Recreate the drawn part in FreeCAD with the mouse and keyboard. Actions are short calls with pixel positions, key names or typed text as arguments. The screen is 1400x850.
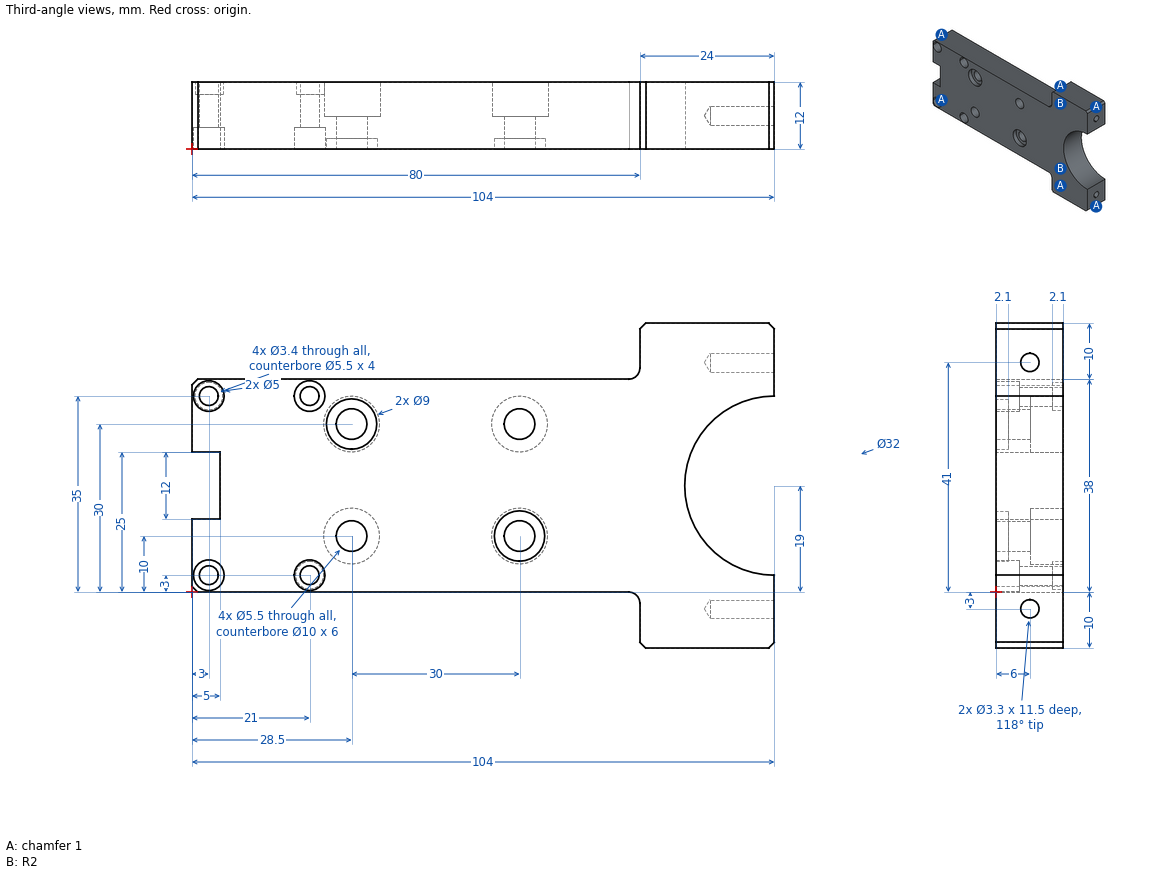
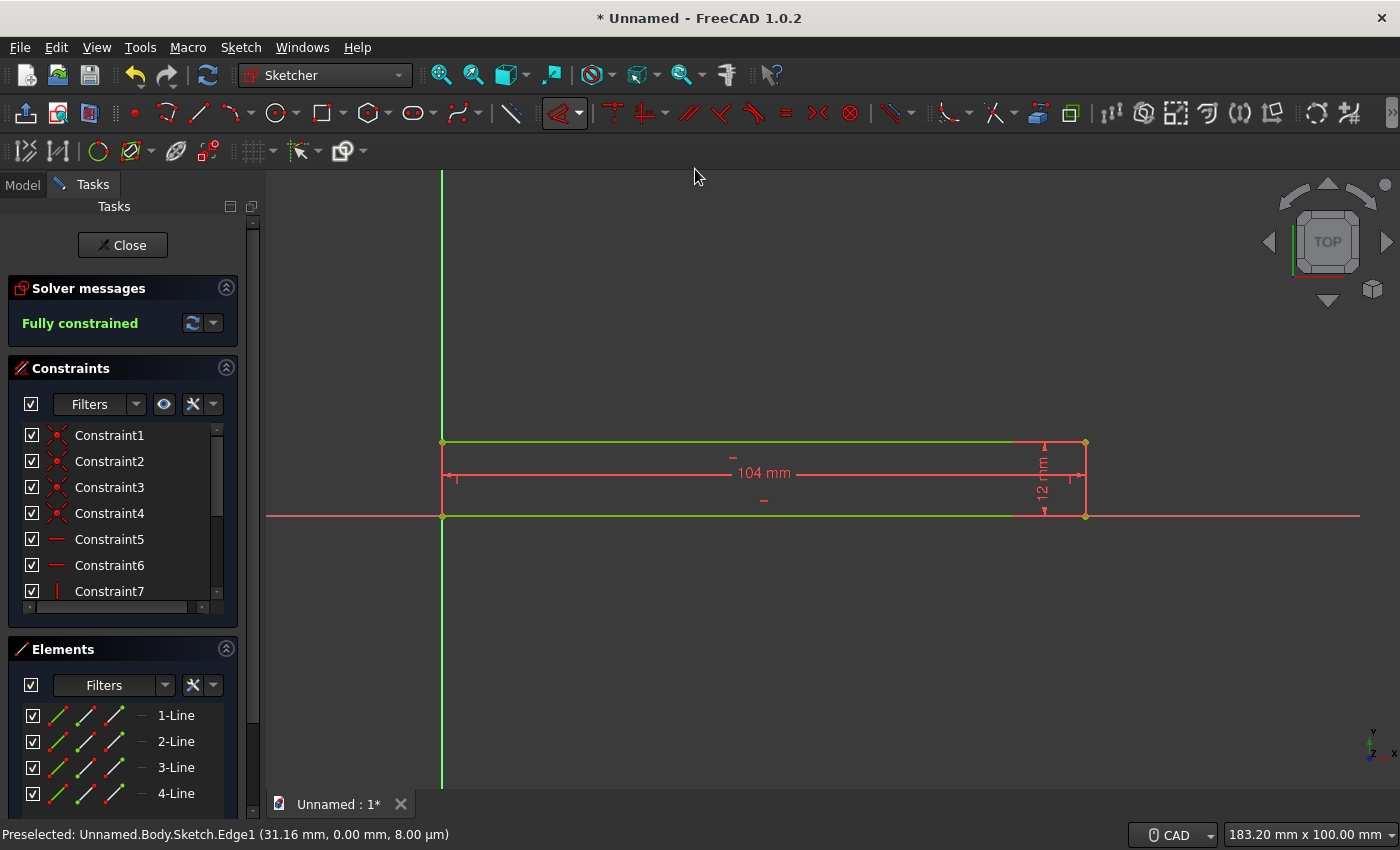
click(123, 245)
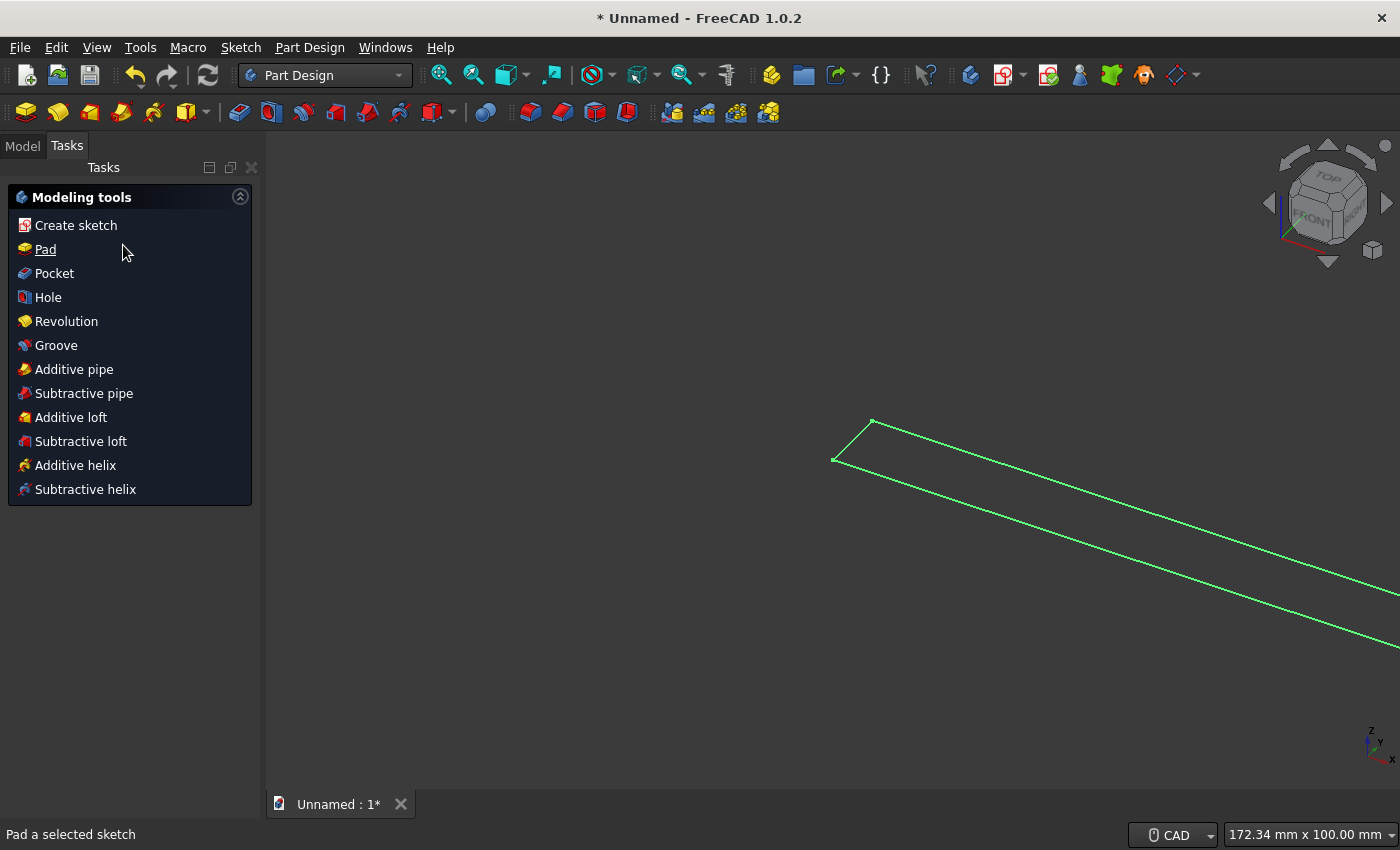
click(26, 112)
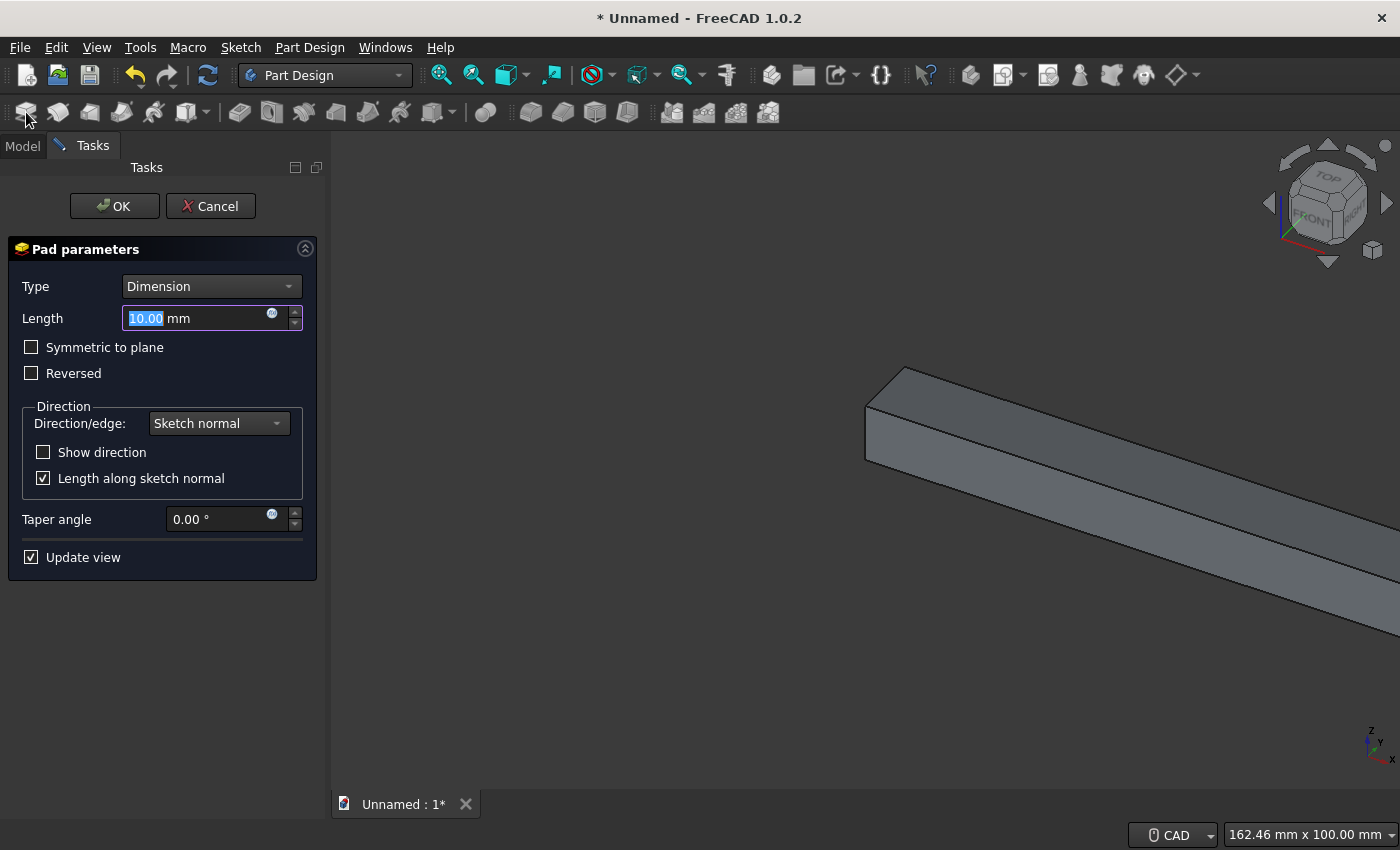
text(38)
key(Tab)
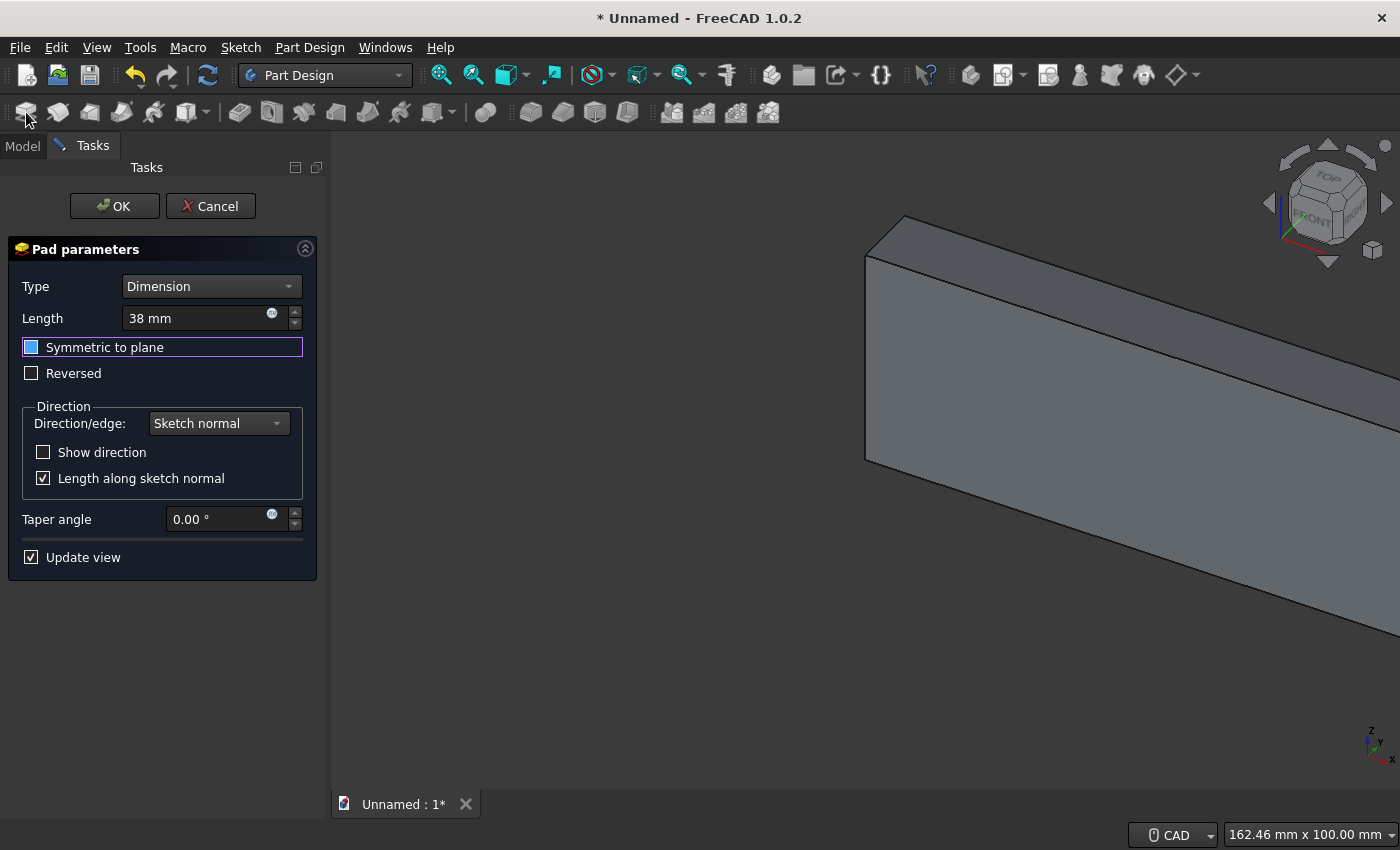
click(115, 206)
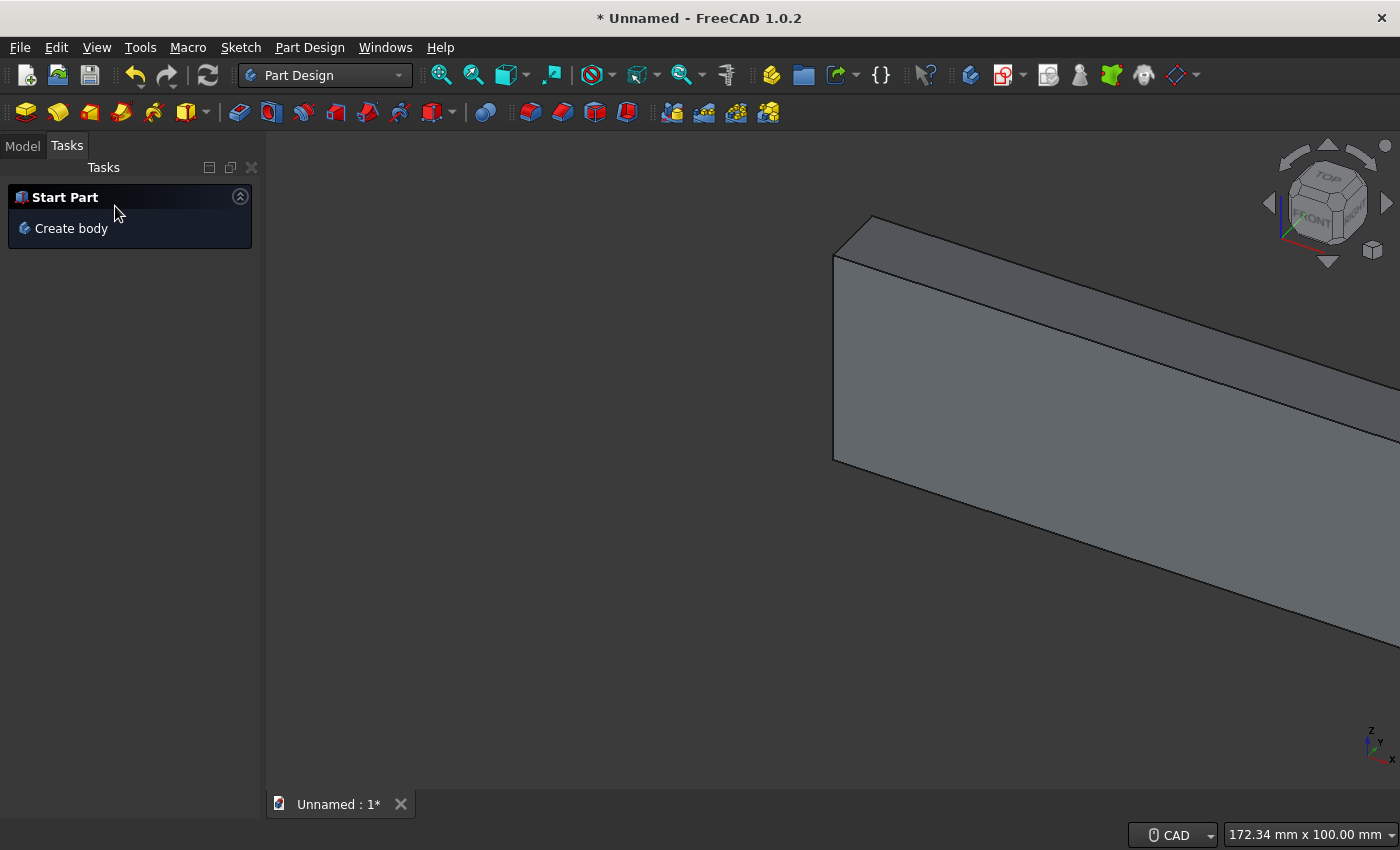
click(442, 76)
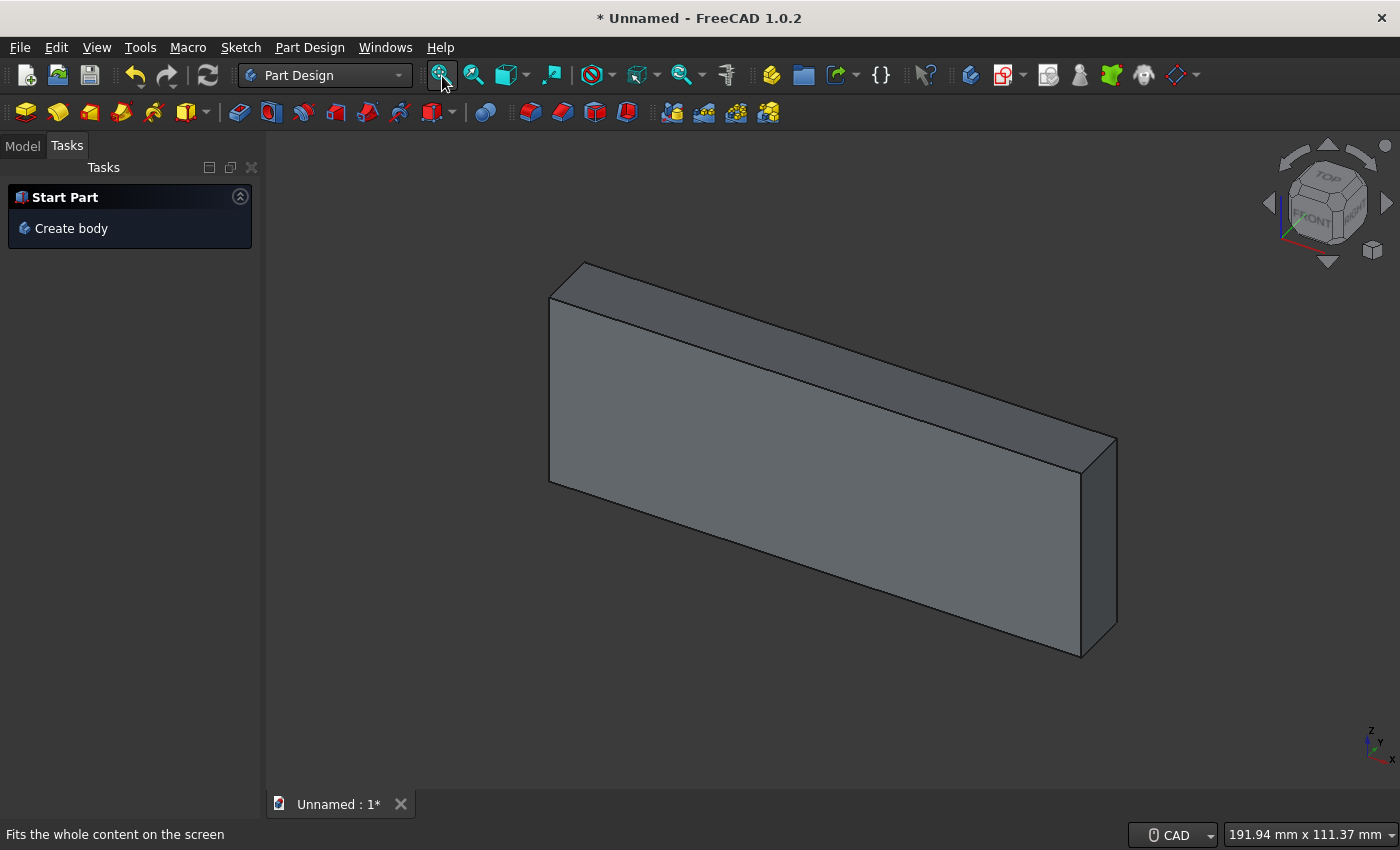
key(4)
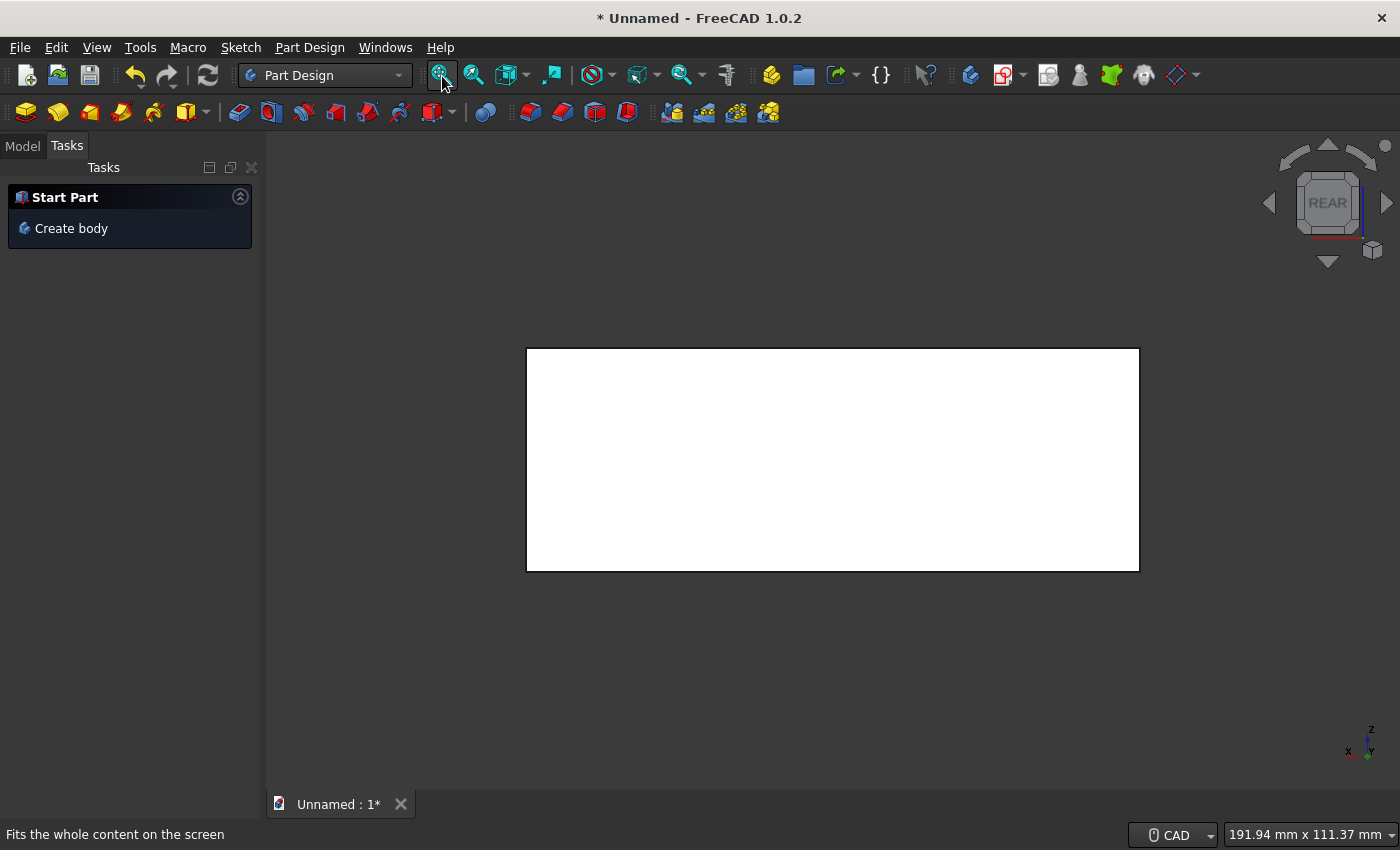
click(657, 459)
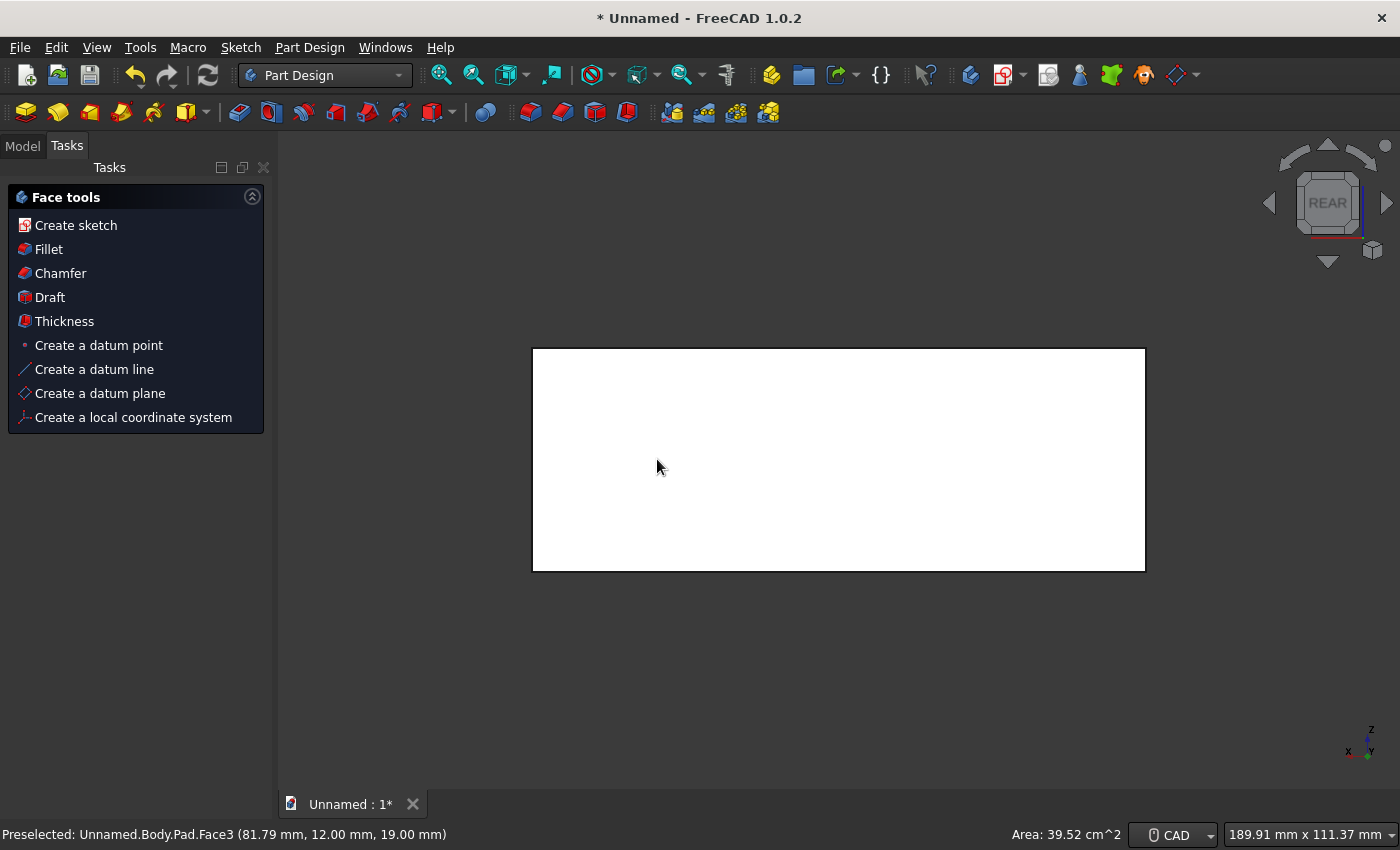
click(1004, 76)